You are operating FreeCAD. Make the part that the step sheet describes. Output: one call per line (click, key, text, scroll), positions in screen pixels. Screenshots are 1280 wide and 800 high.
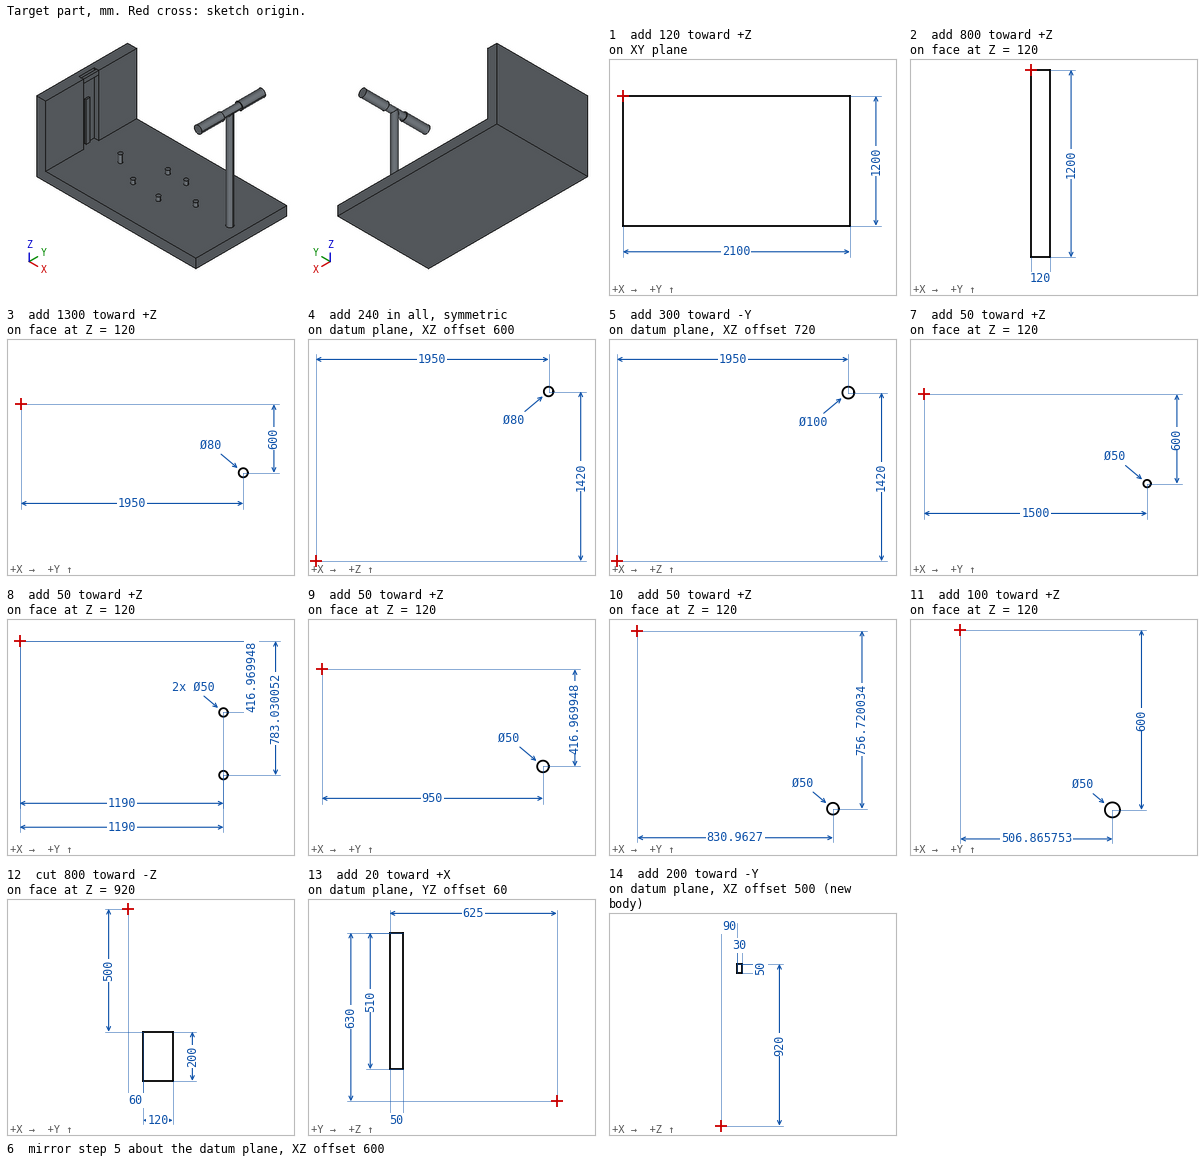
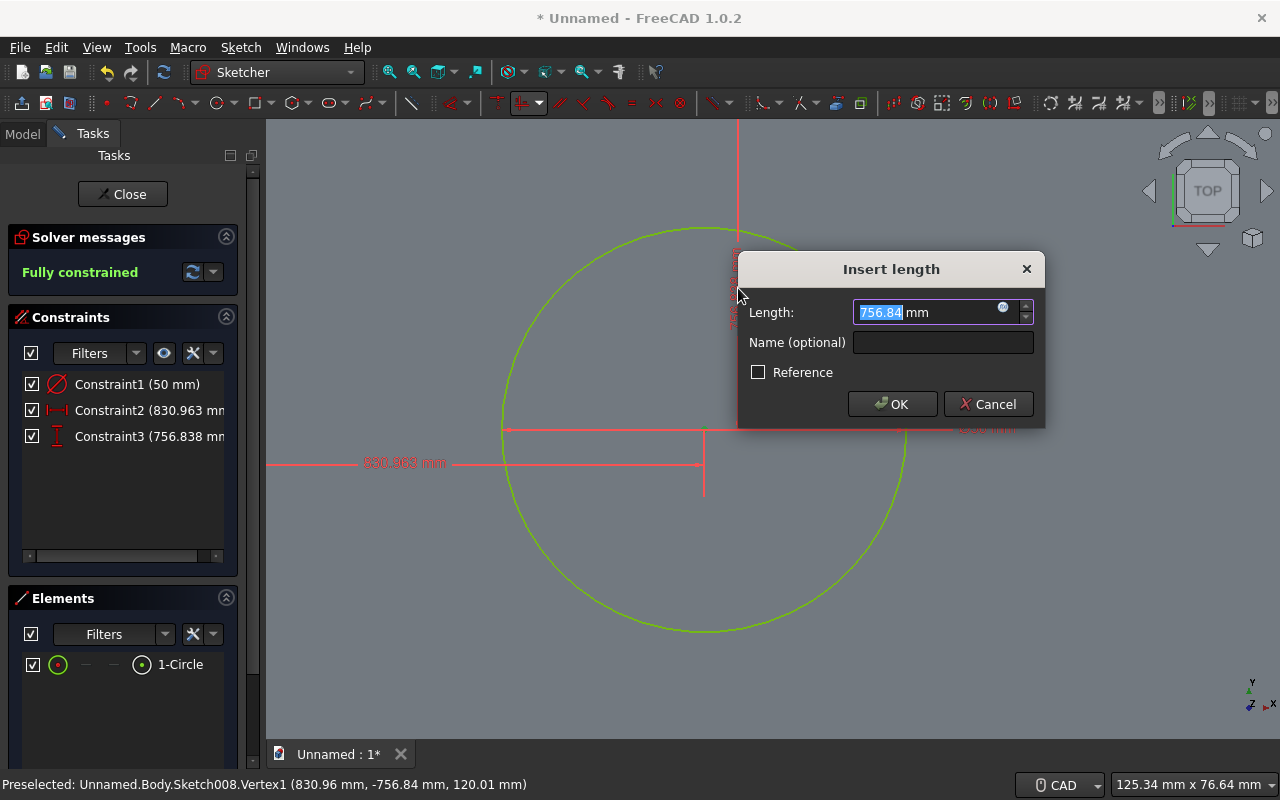
text(756.720034)
key(Return)
key(Escape)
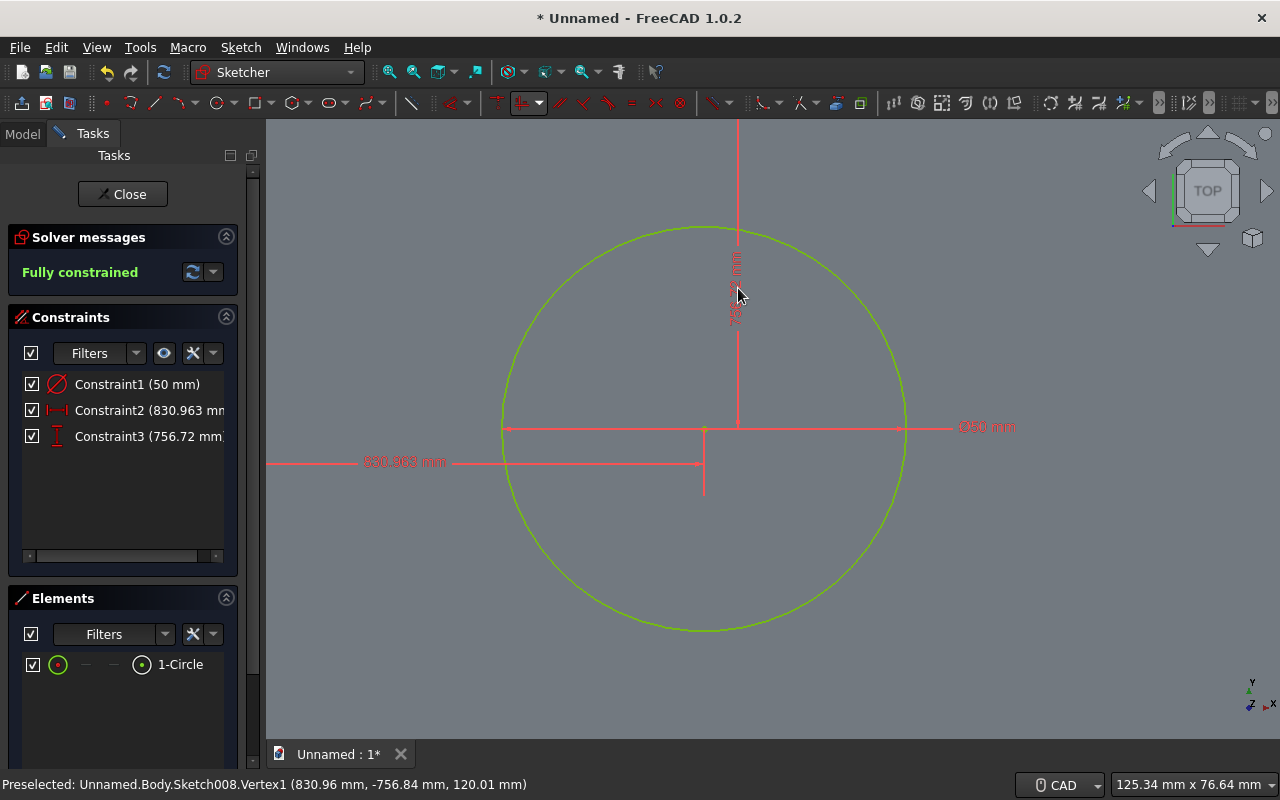
click(123, 194)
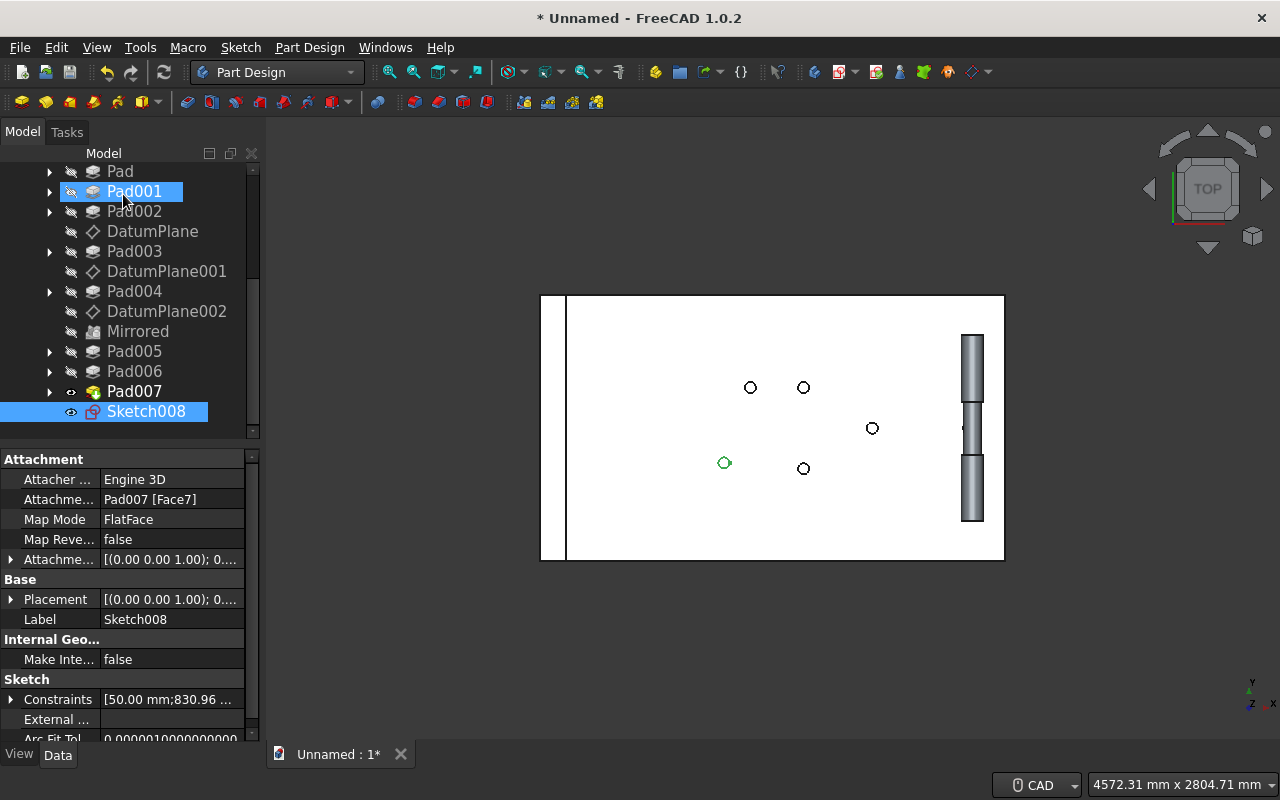
click(22, 102)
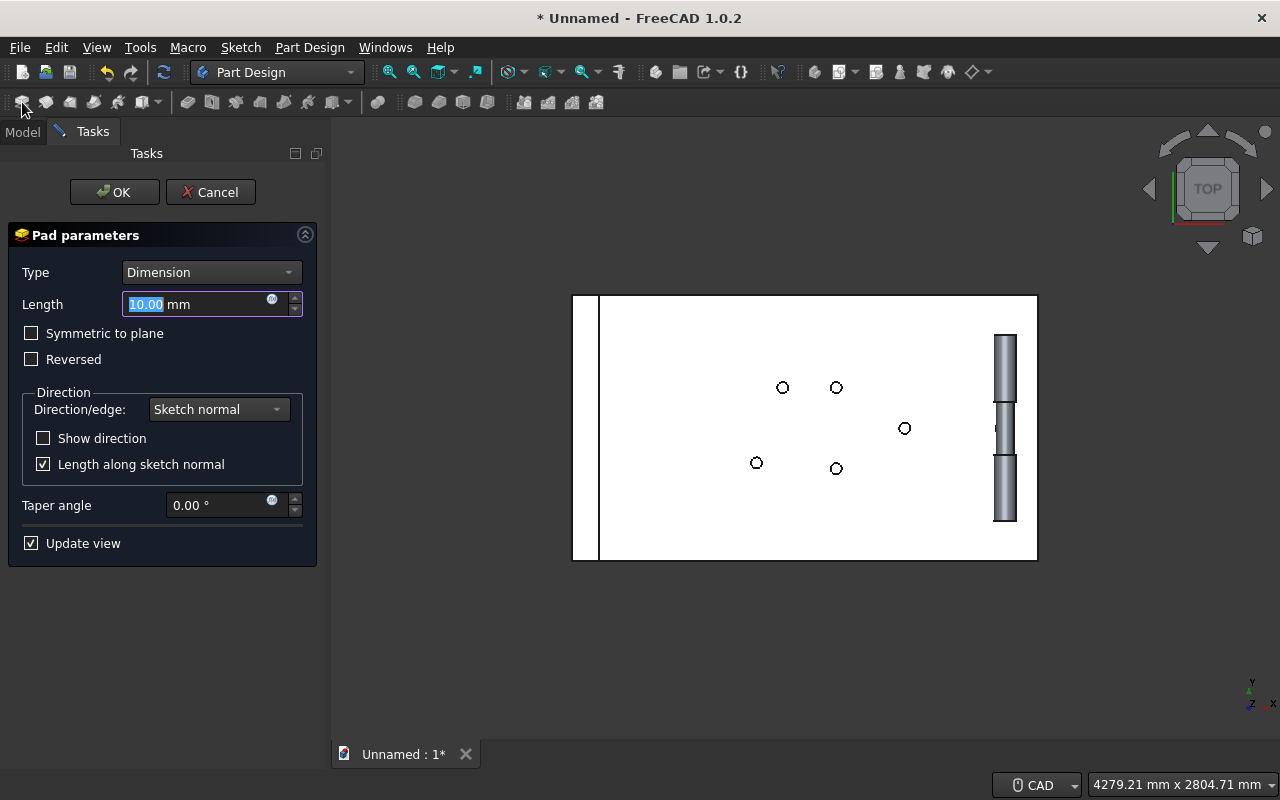
text(50)
key(Tab)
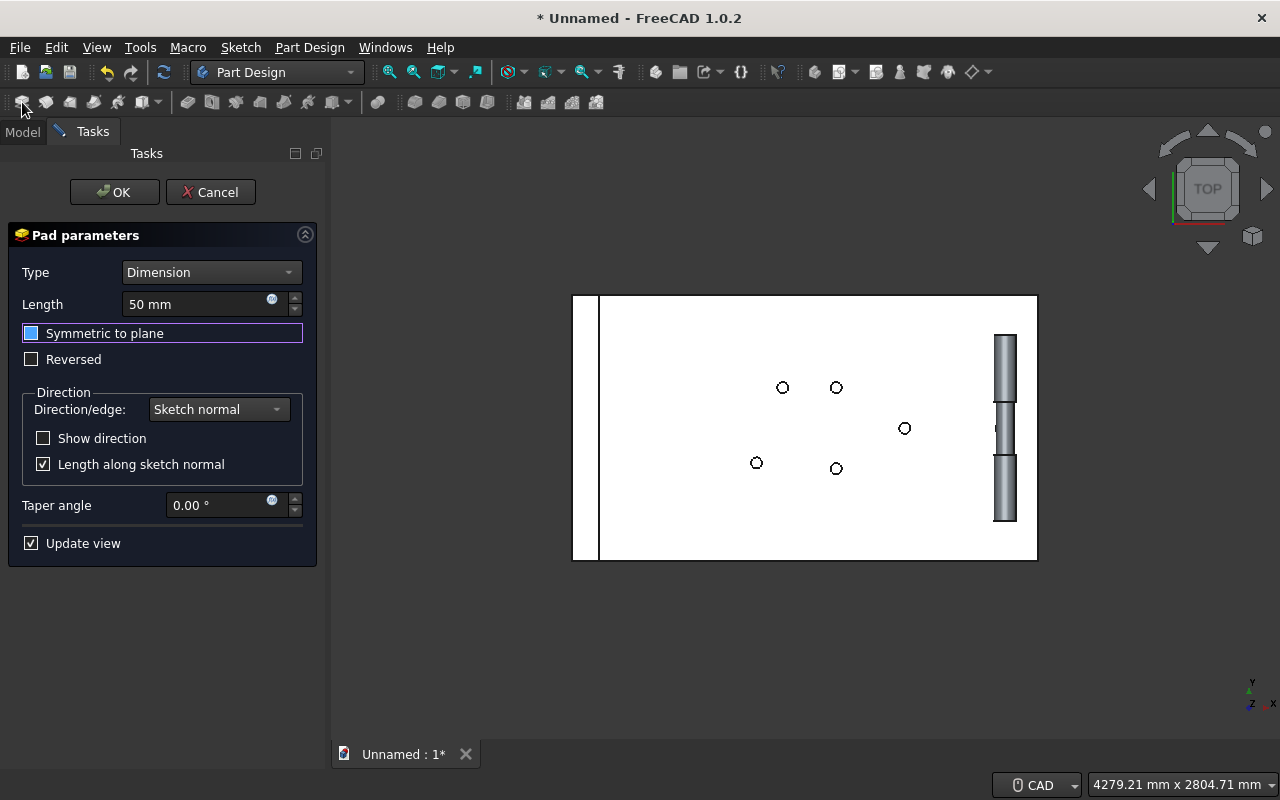
click(115, 192)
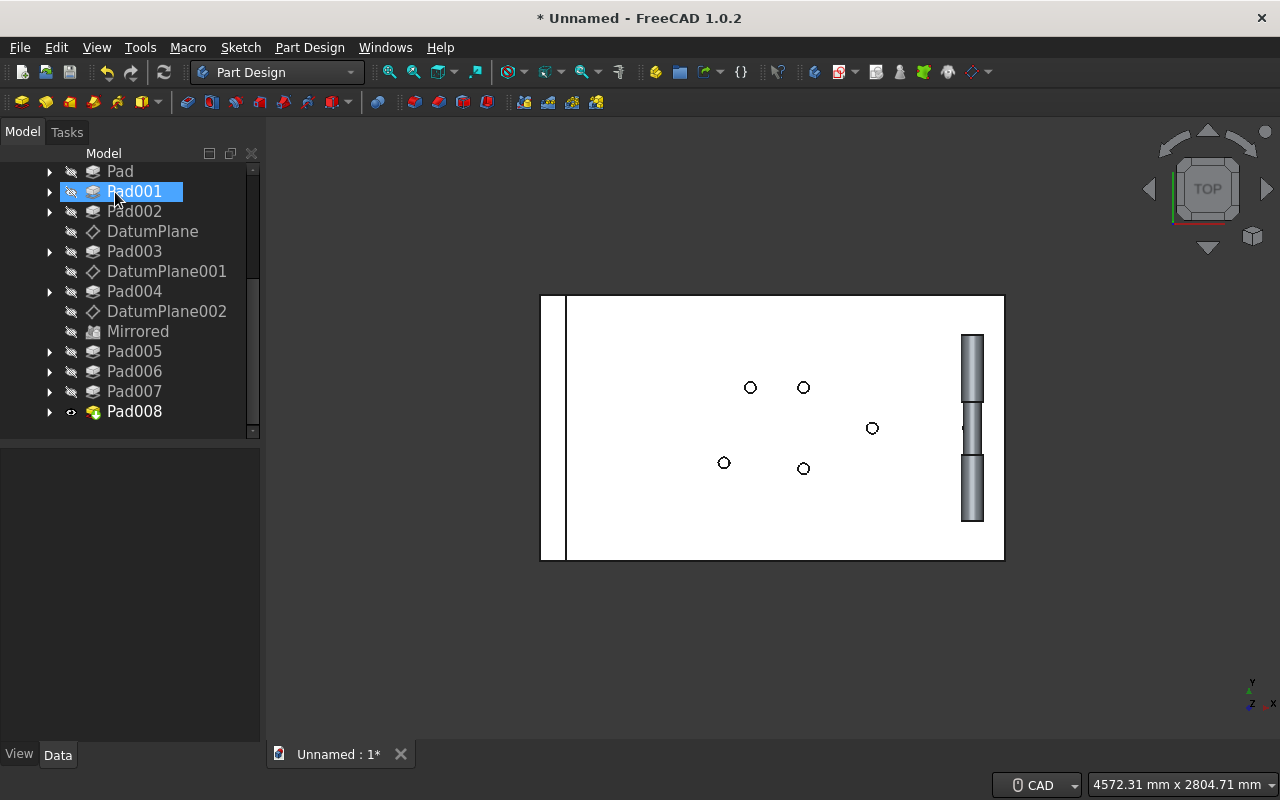
click(660, 389)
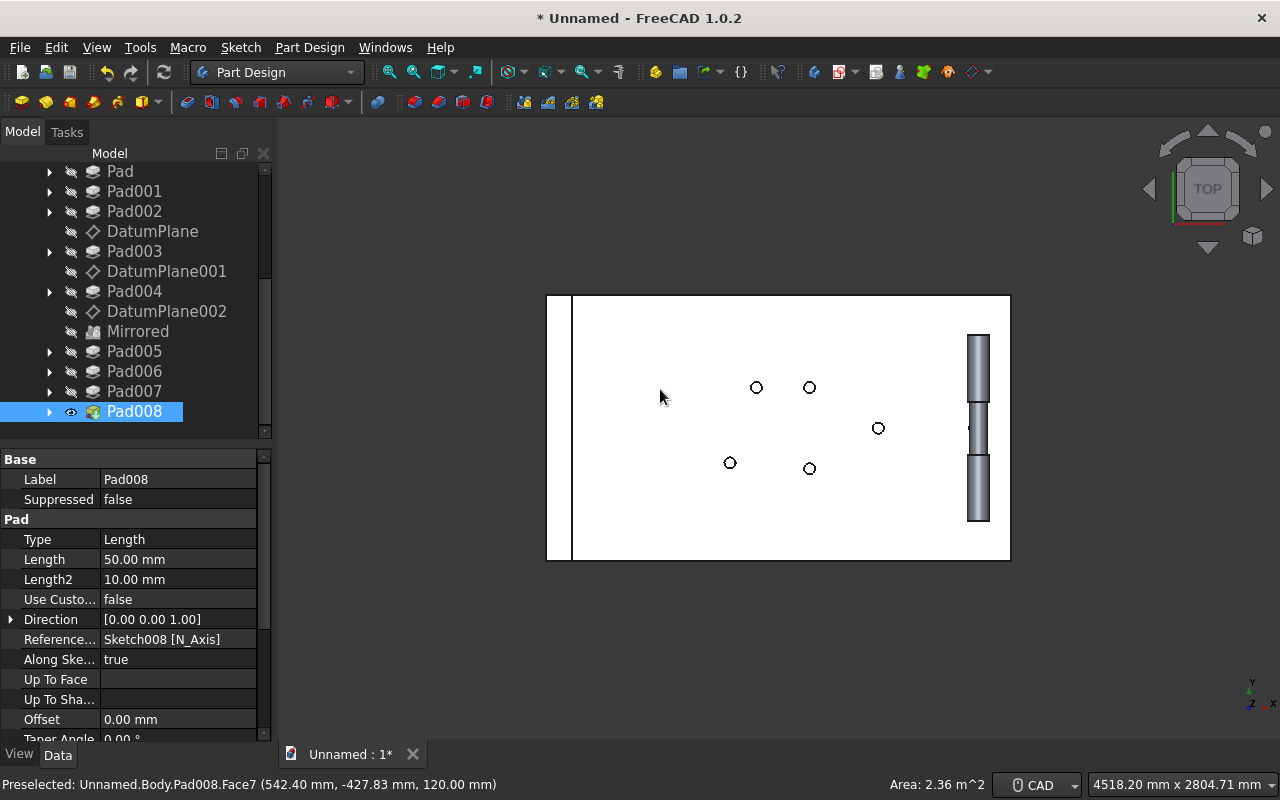
click(840, 72)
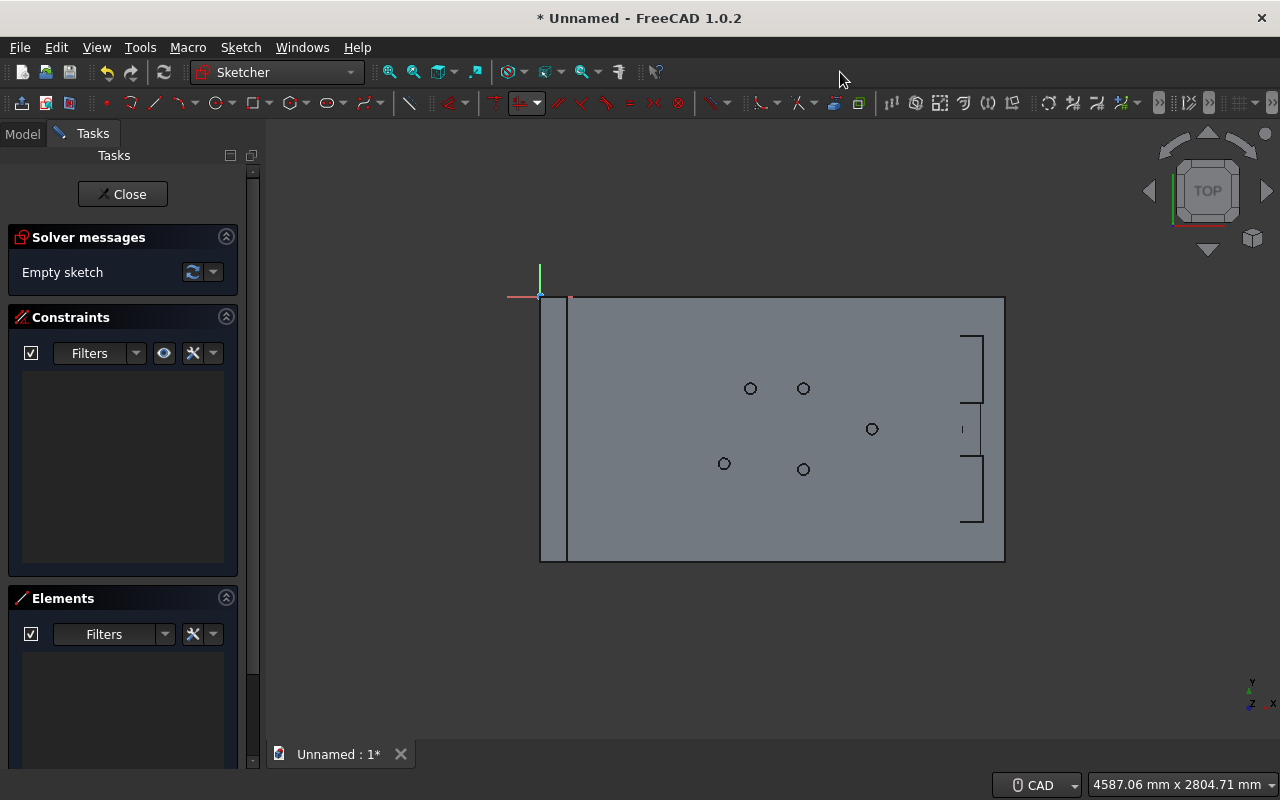
scroll(650, 429, up, 15)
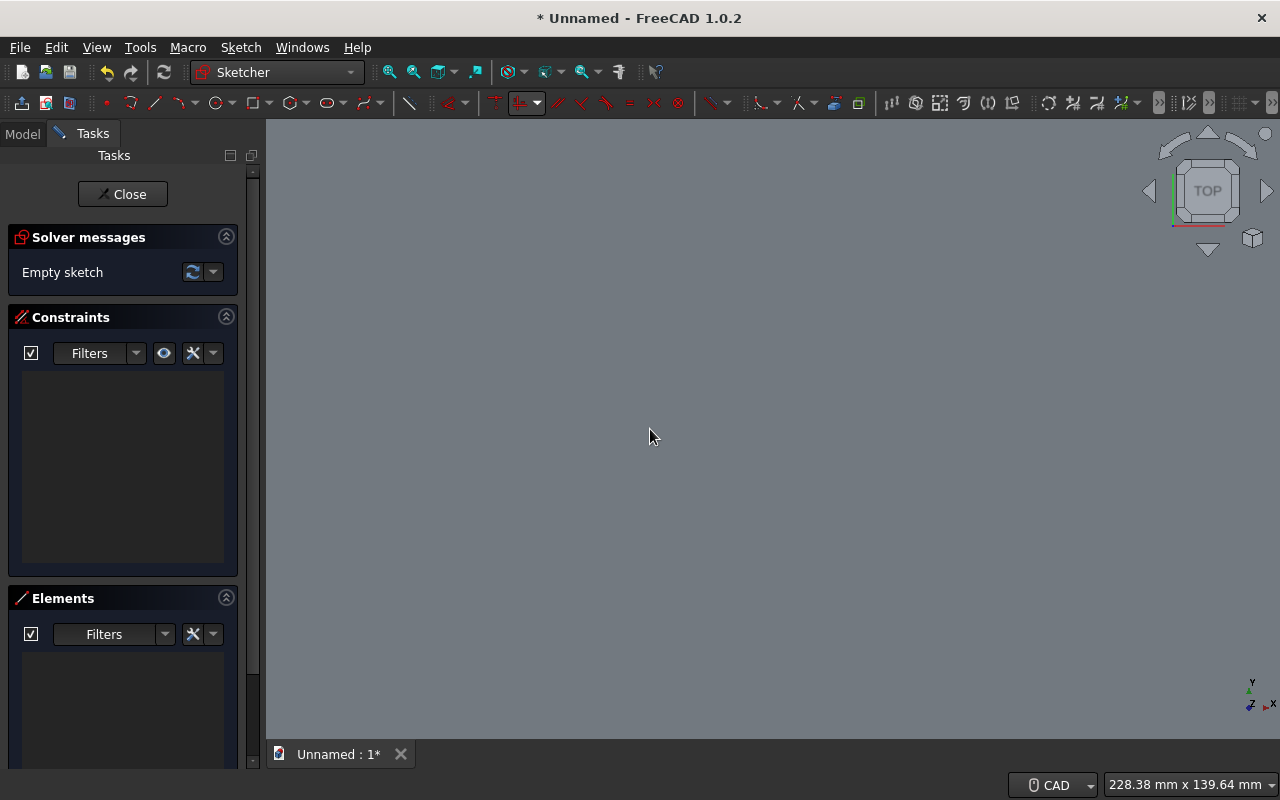
scroll(679, 416, up, 3)